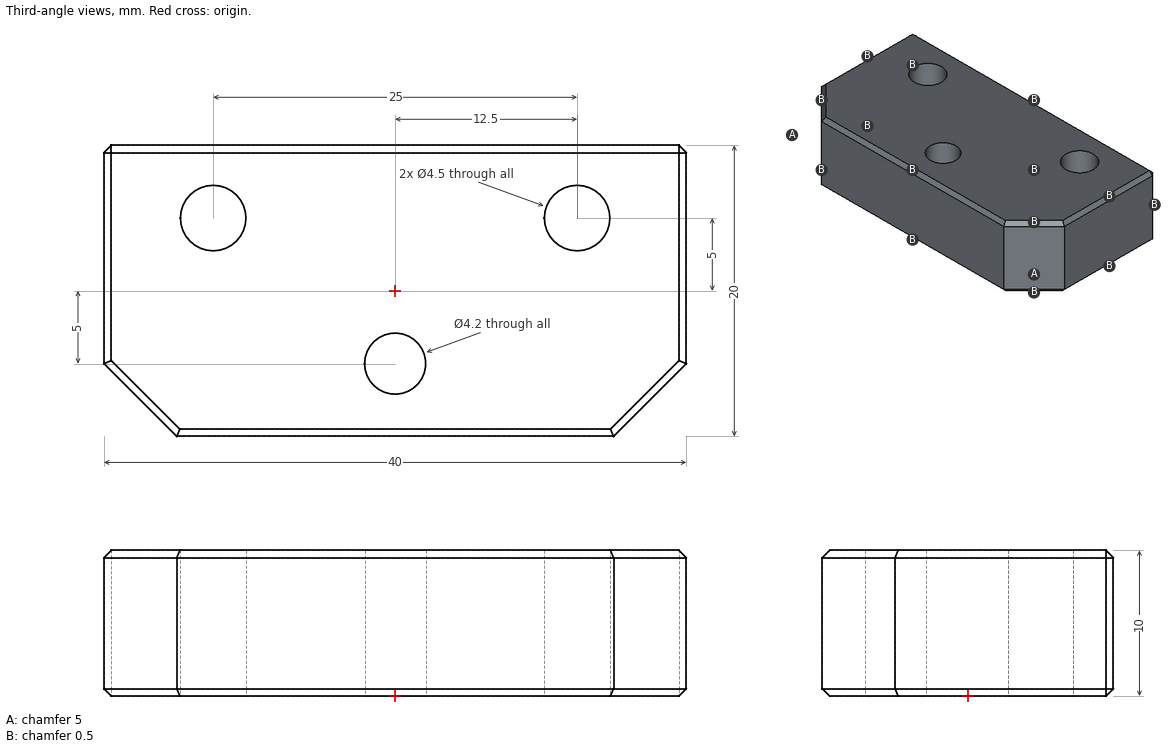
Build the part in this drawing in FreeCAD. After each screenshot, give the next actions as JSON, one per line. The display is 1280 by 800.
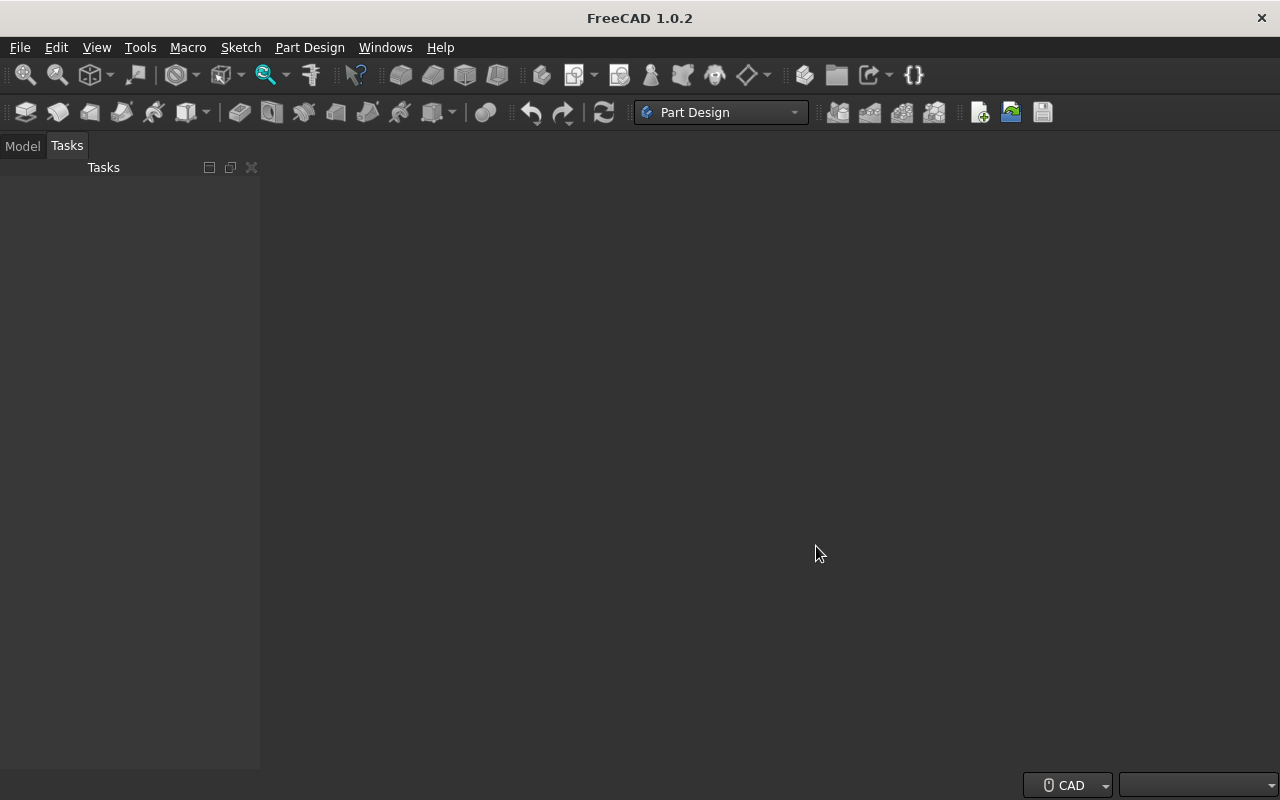
{"action": "key", "text": "ctrl+n"}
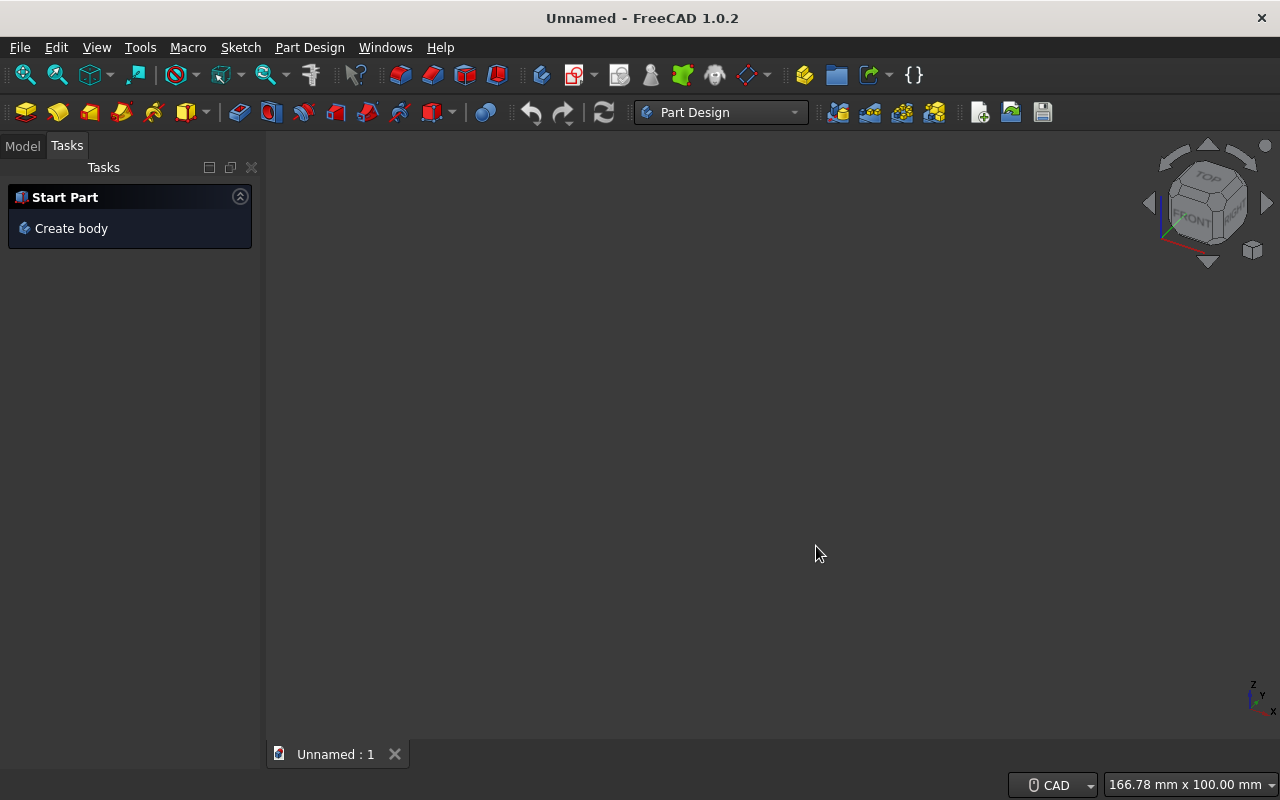
{"action": "left_click", "coordinate": [574, 76]}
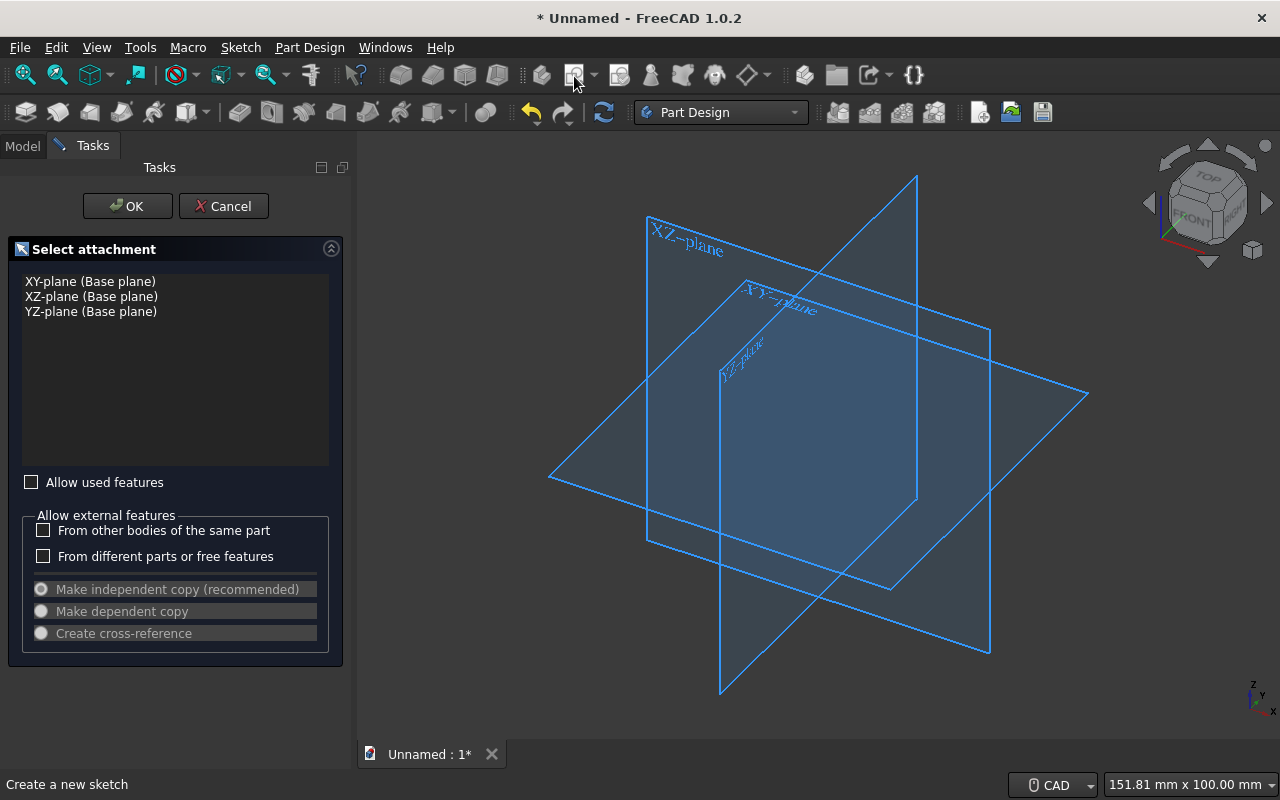
{"action": "left_click", "coordinate": [82, 282]}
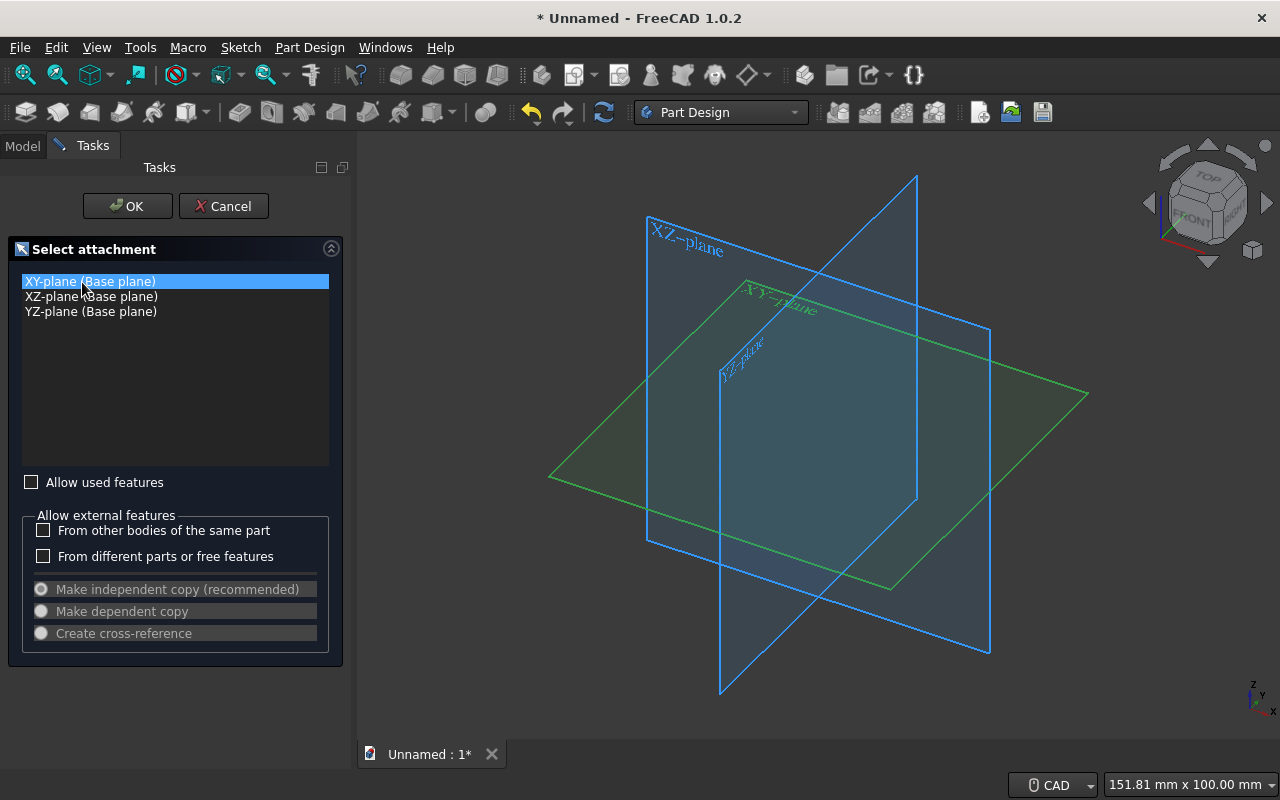
{"action": "left_click", "coordinate": [128, 206]}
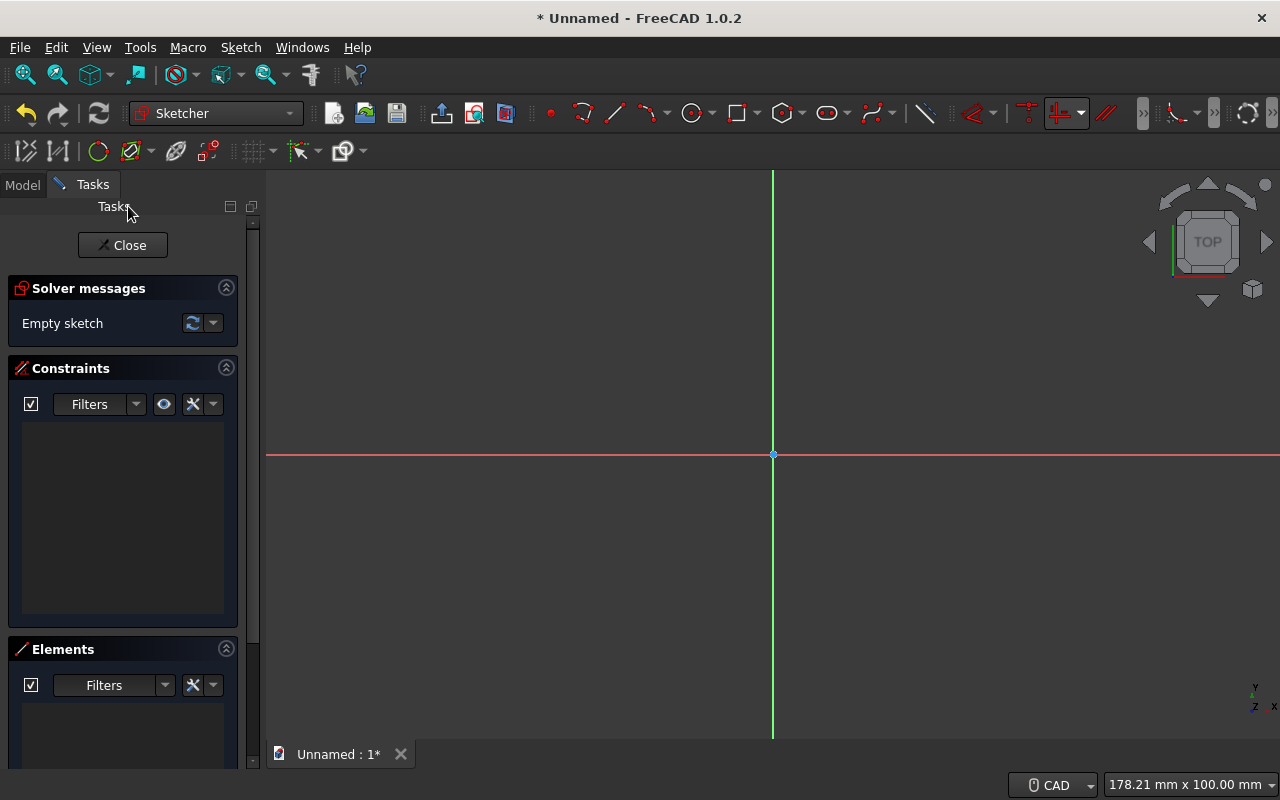
{"action": "scroll", "coordinate": [813, 454], "scroll_direction": "up", "scroll_amount": 5}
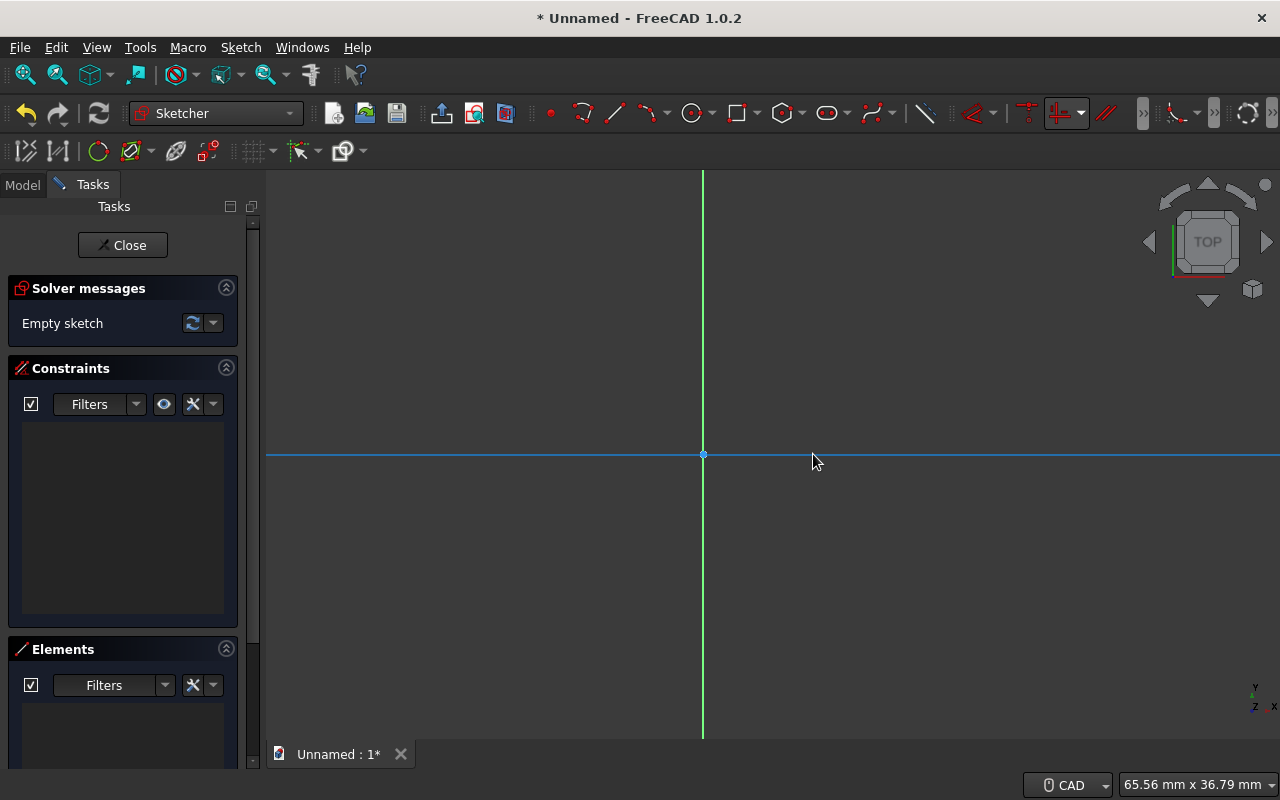
{"action": "key", "text": "g v"}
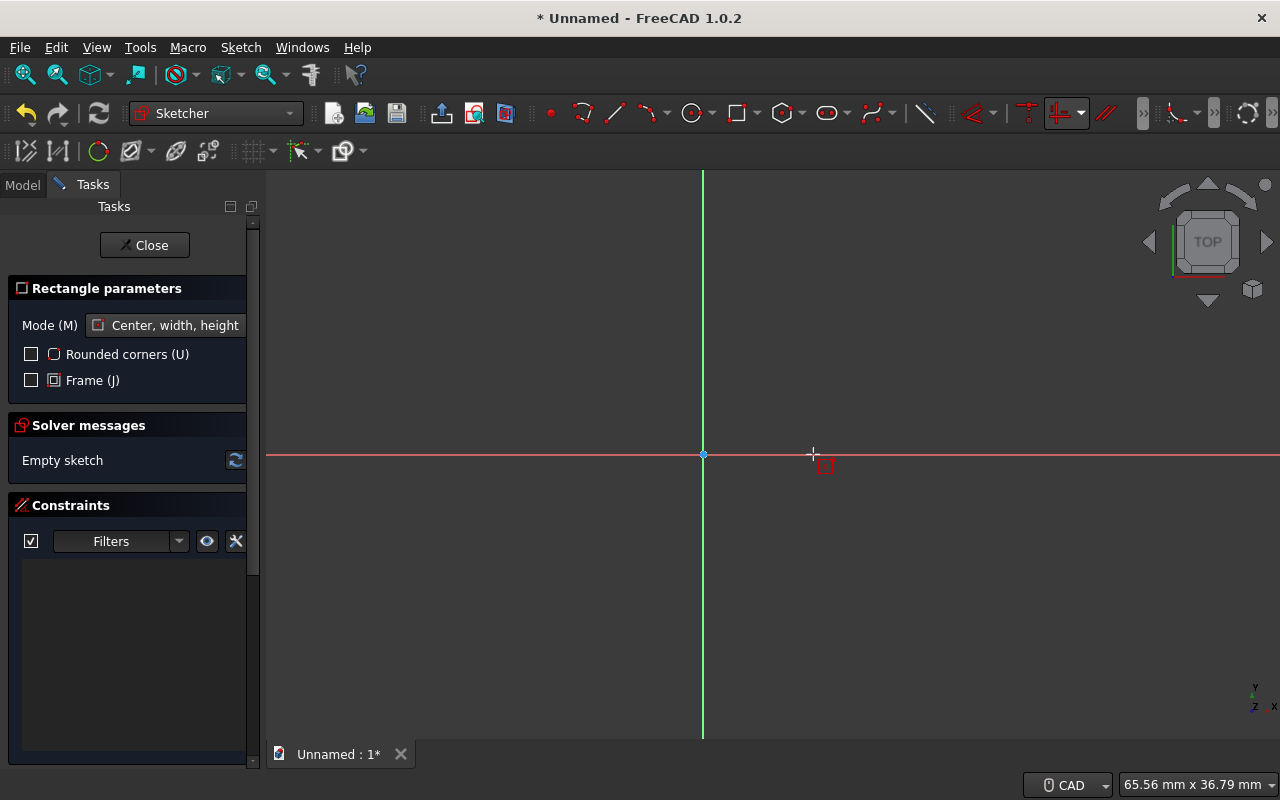
{"action": "left_click", "coordinate": [703, 454]}
{"action": "mouse_move", "coordinate": [1013, 300]}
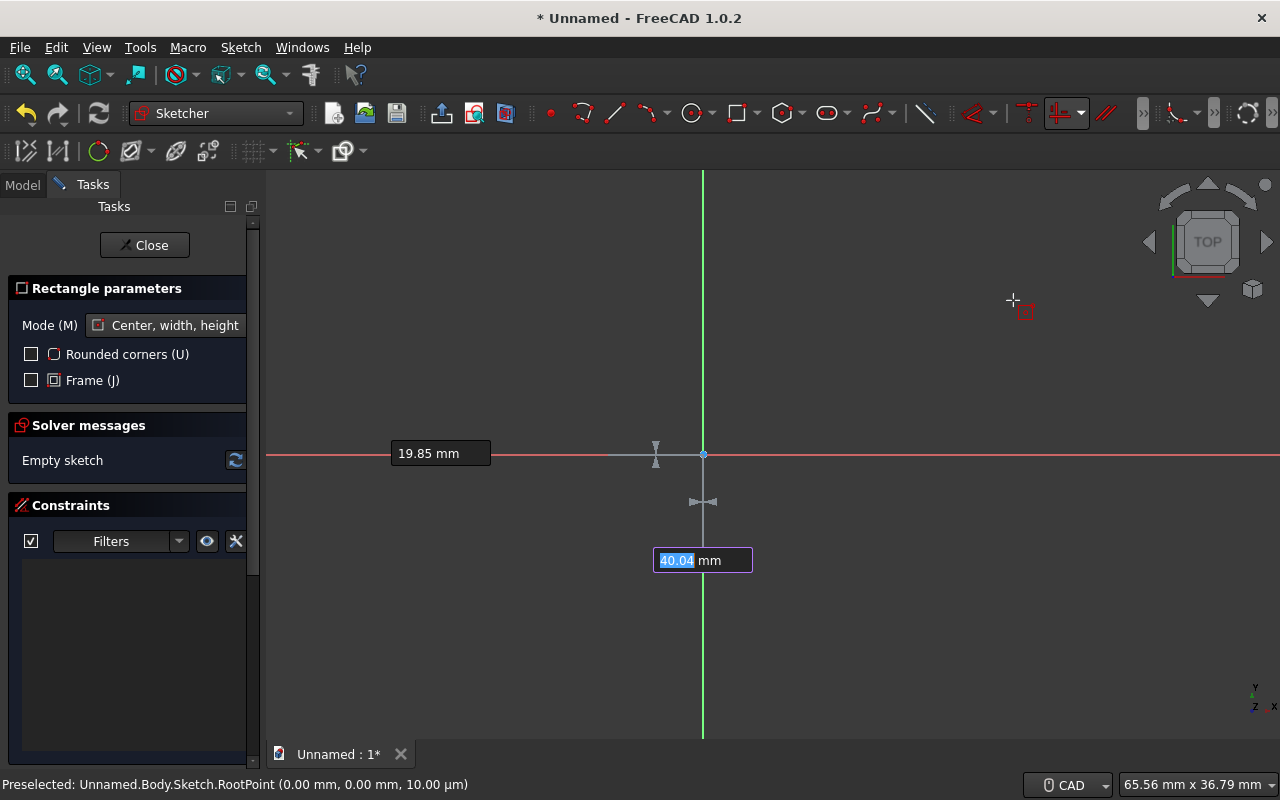
{"action": "type", "text": "40"}
{"action": "key", "text": "Tab"}
{"action": "type", "text": "20"}
{"action": "key", "text": "Return"}
{"action": "key", "text": "Escape"}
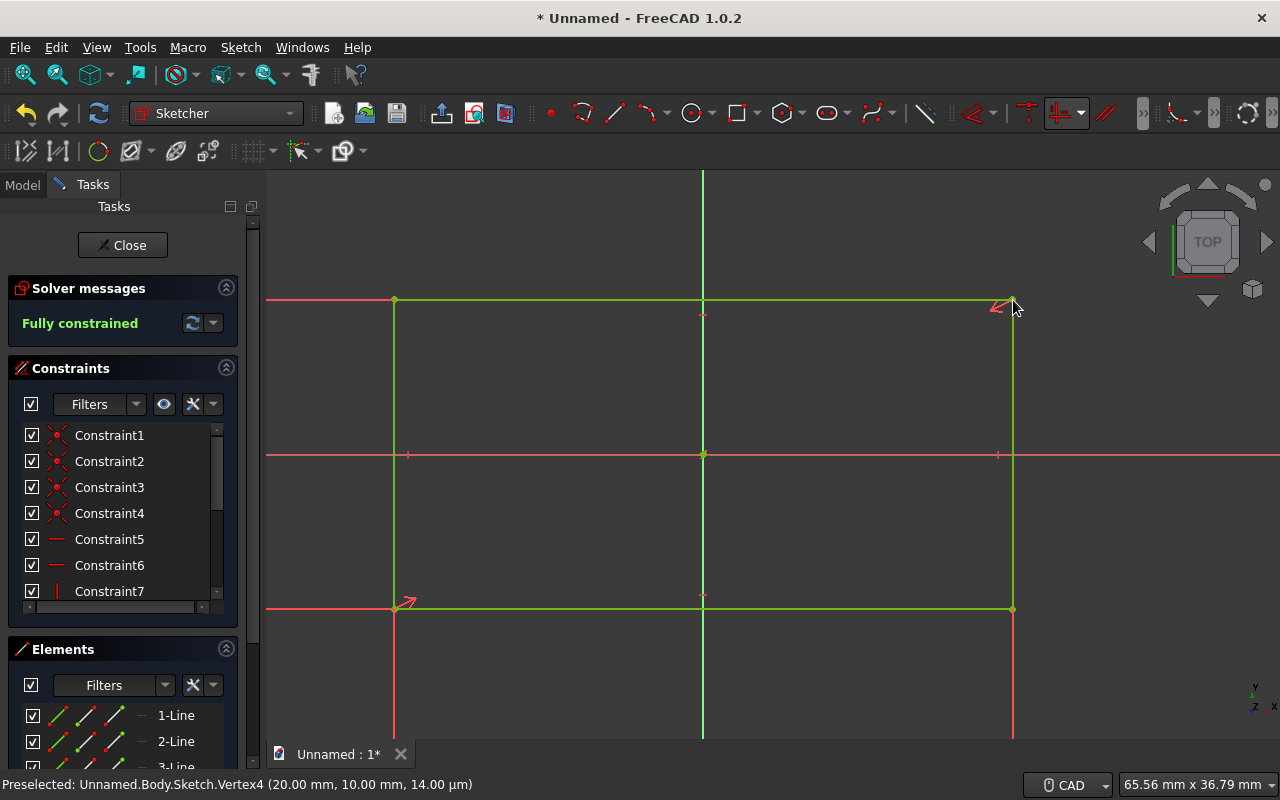
{"action": "left_click", "coordinate": [123, 245]}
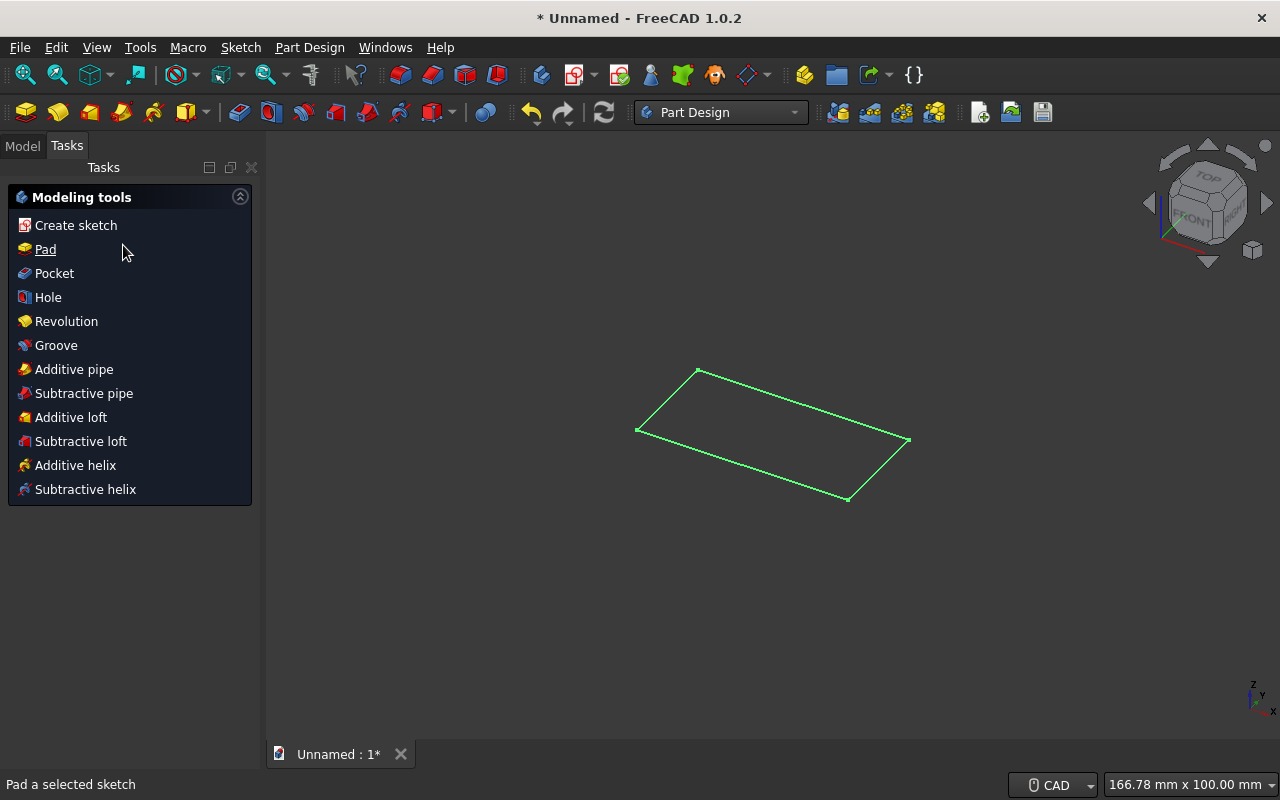
{"action": "left_click", "coordinate": [26, 112]}